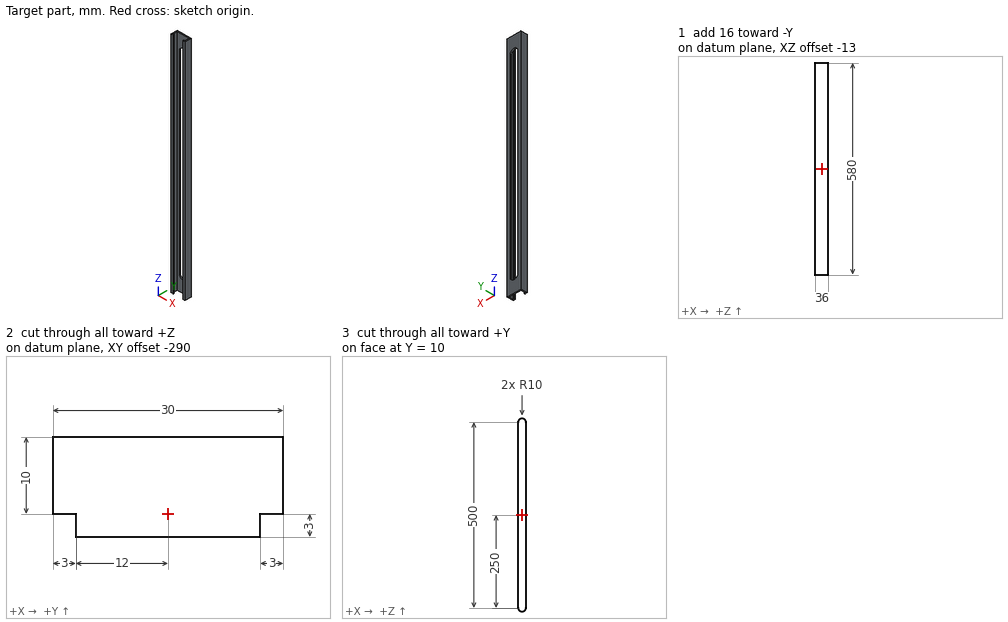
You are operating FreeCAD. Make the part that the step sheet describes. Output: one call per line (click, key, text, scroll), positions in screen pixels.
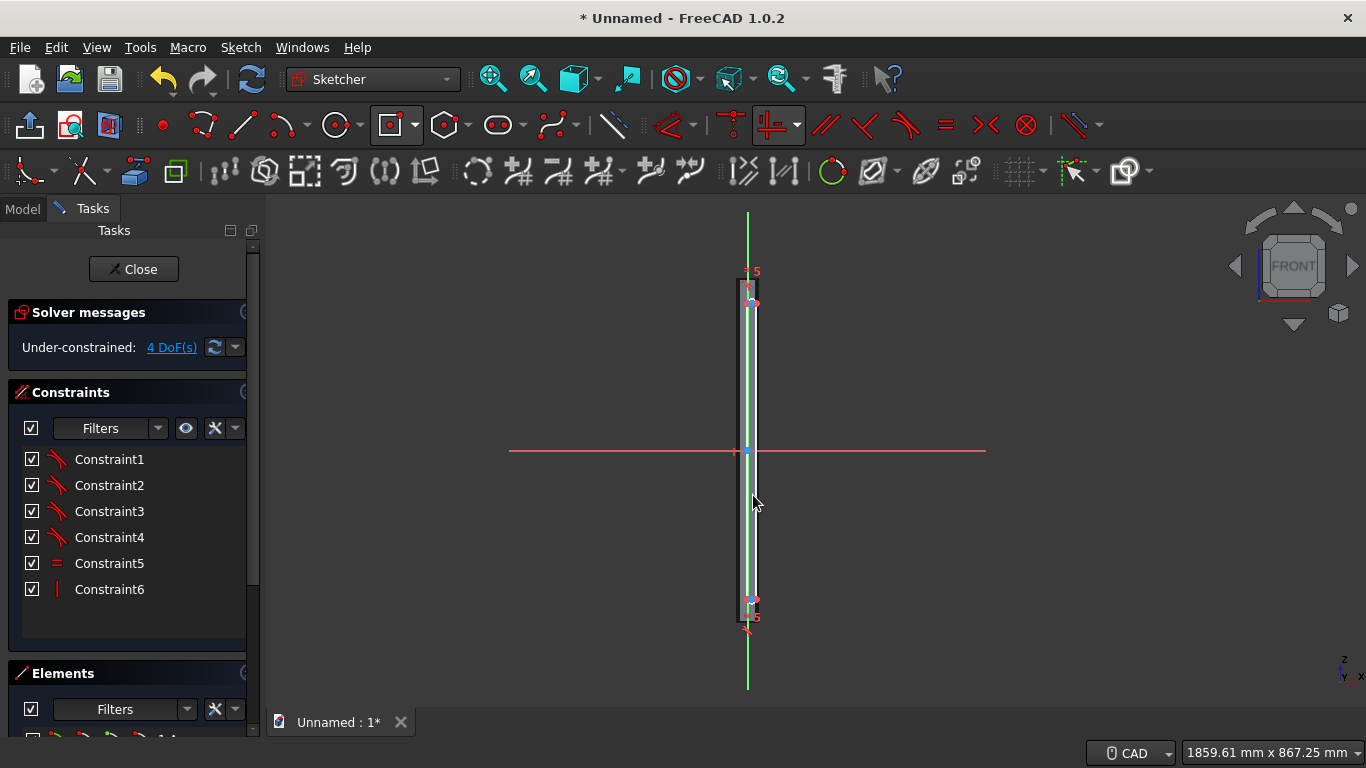
scroll(752, 599, up, 6)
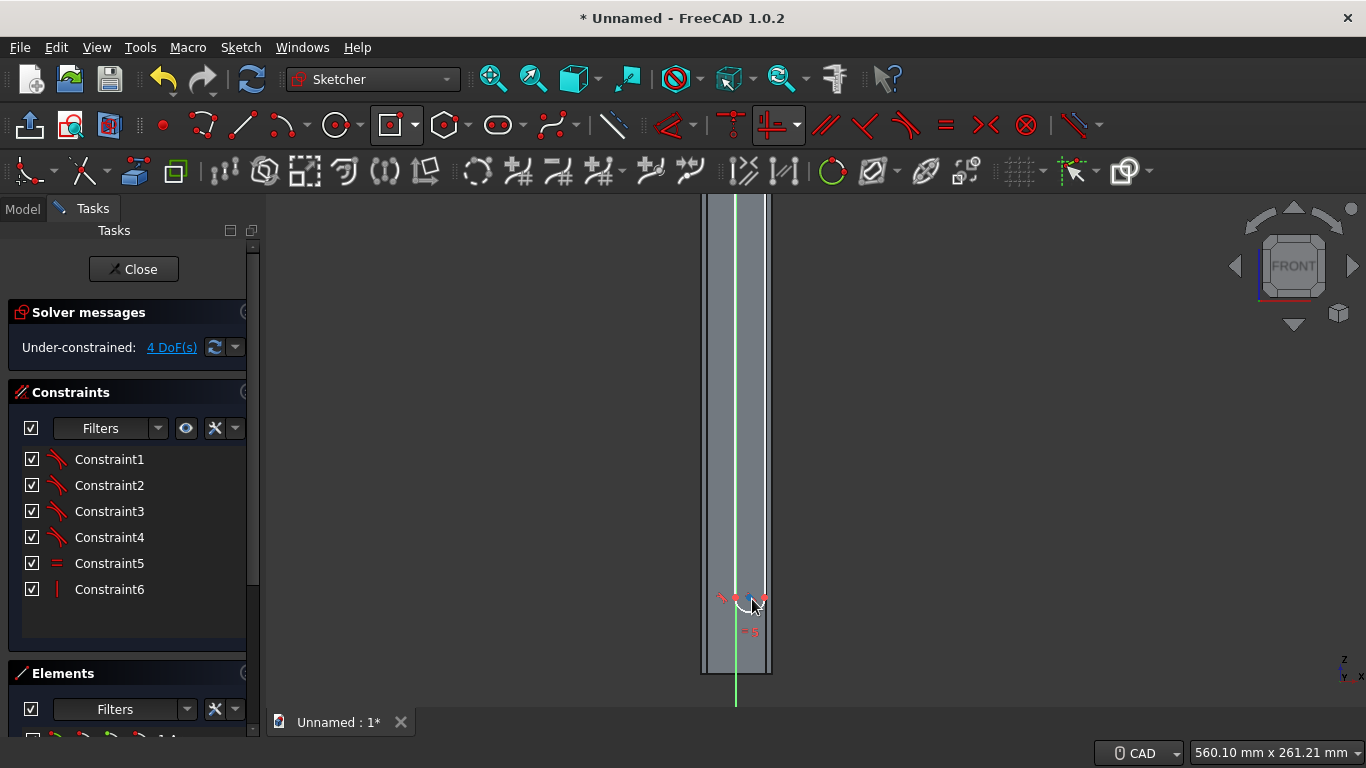
click(750, 598)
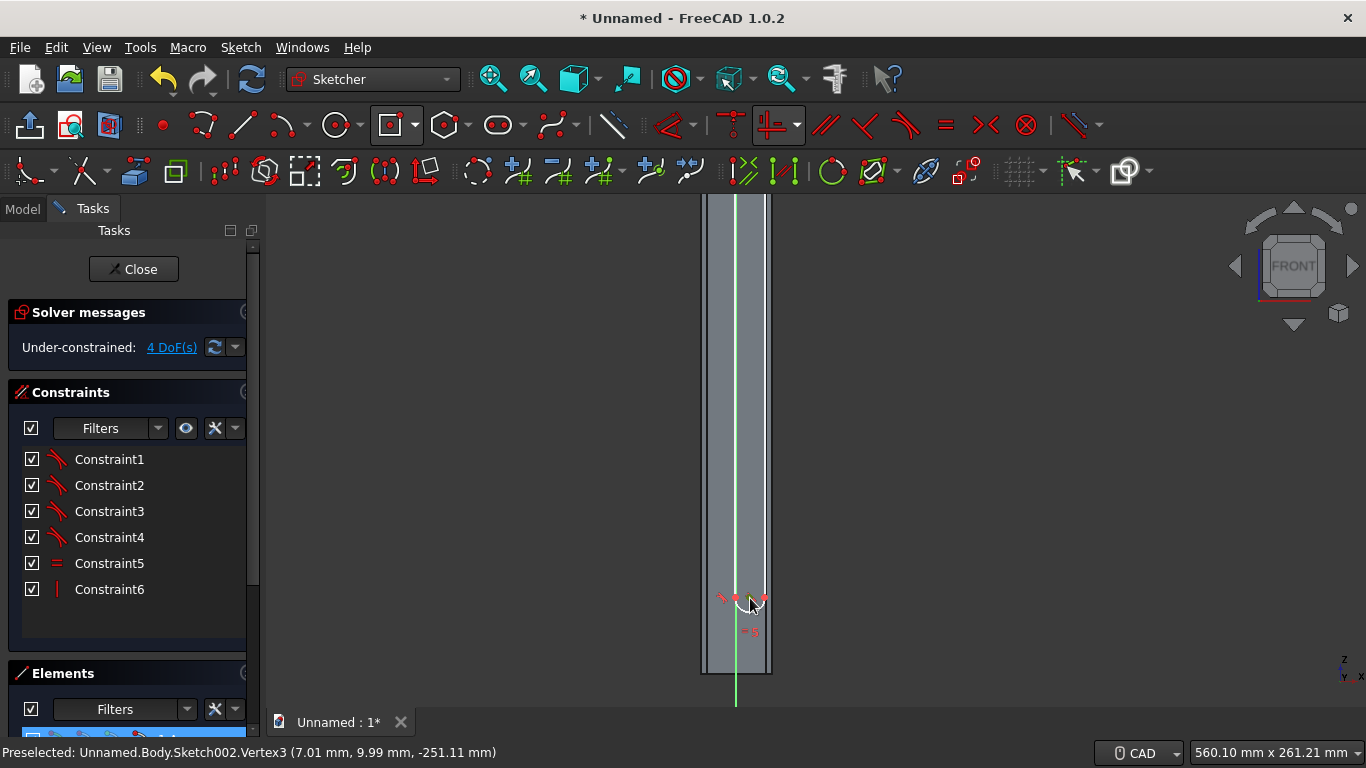
click(736, 646)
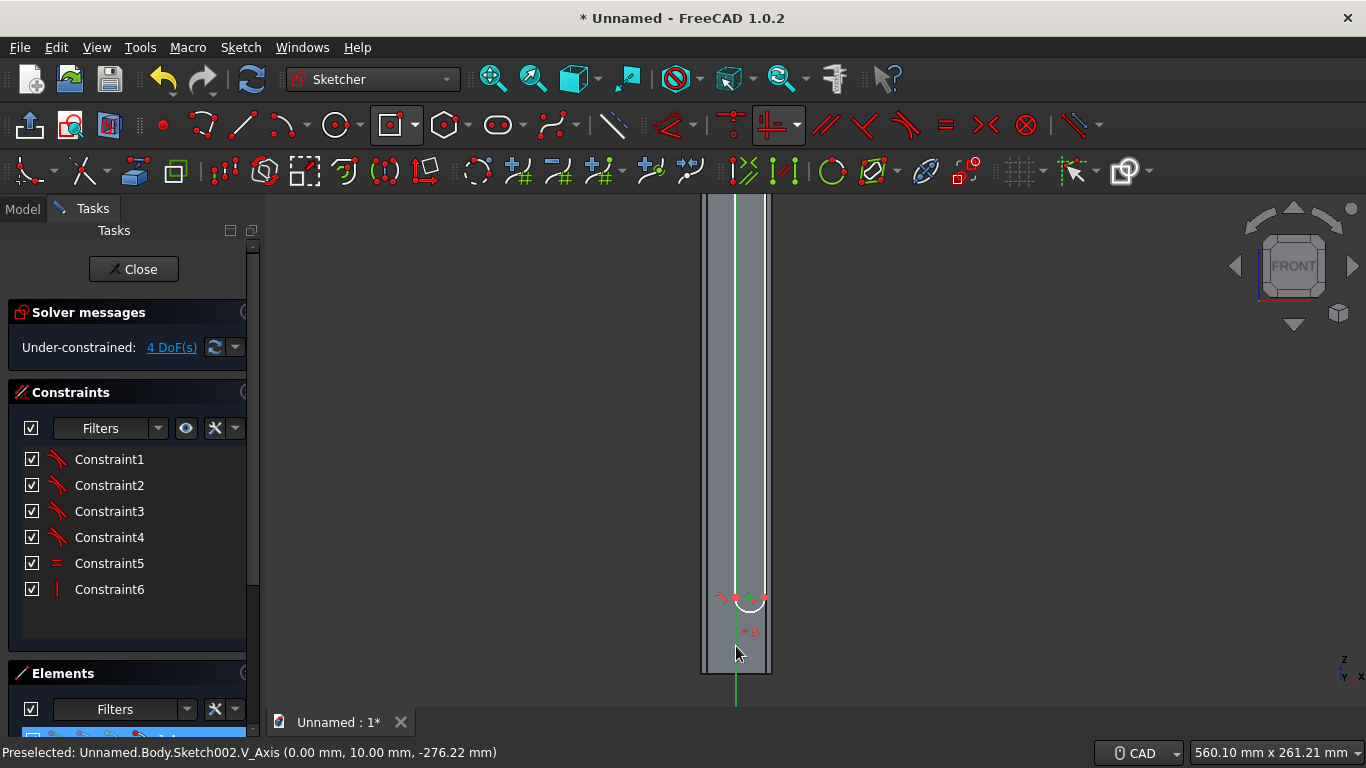
click(732, 126)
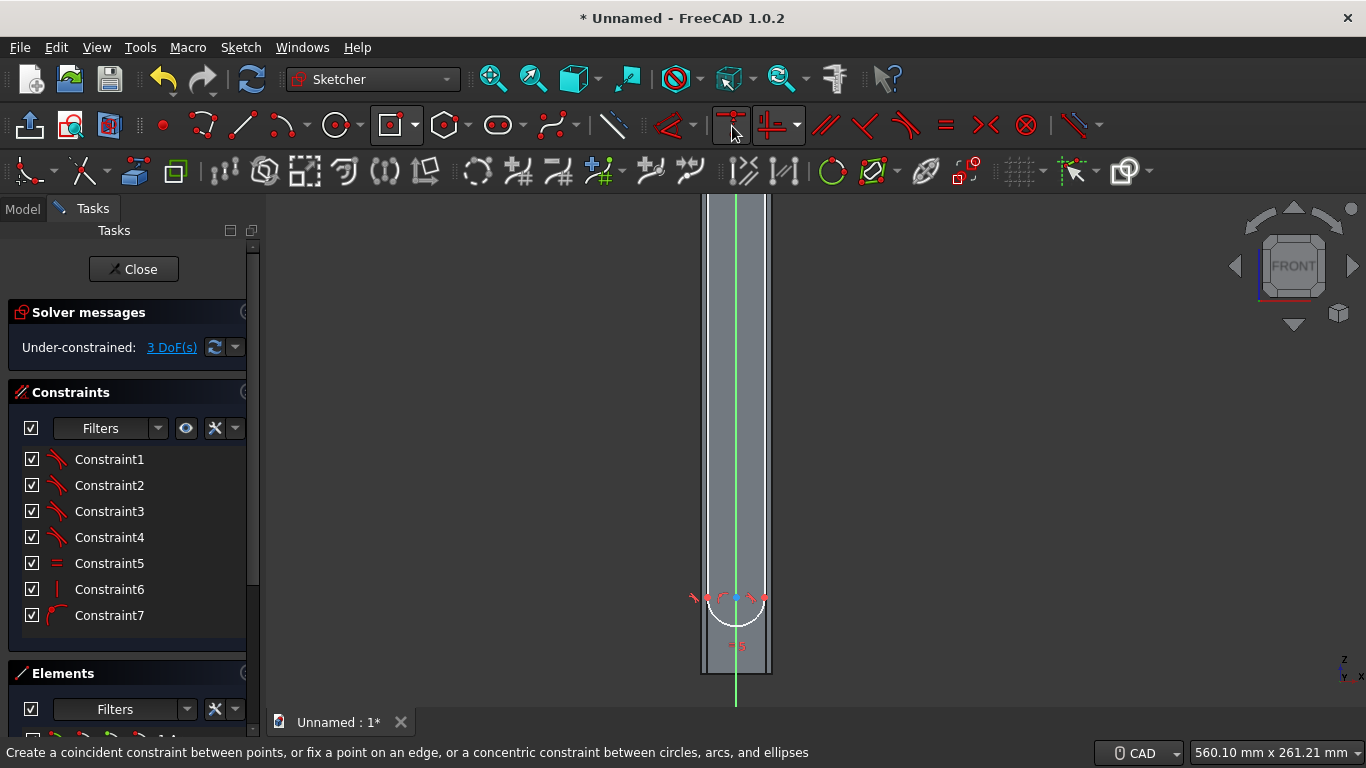
click(668, 126)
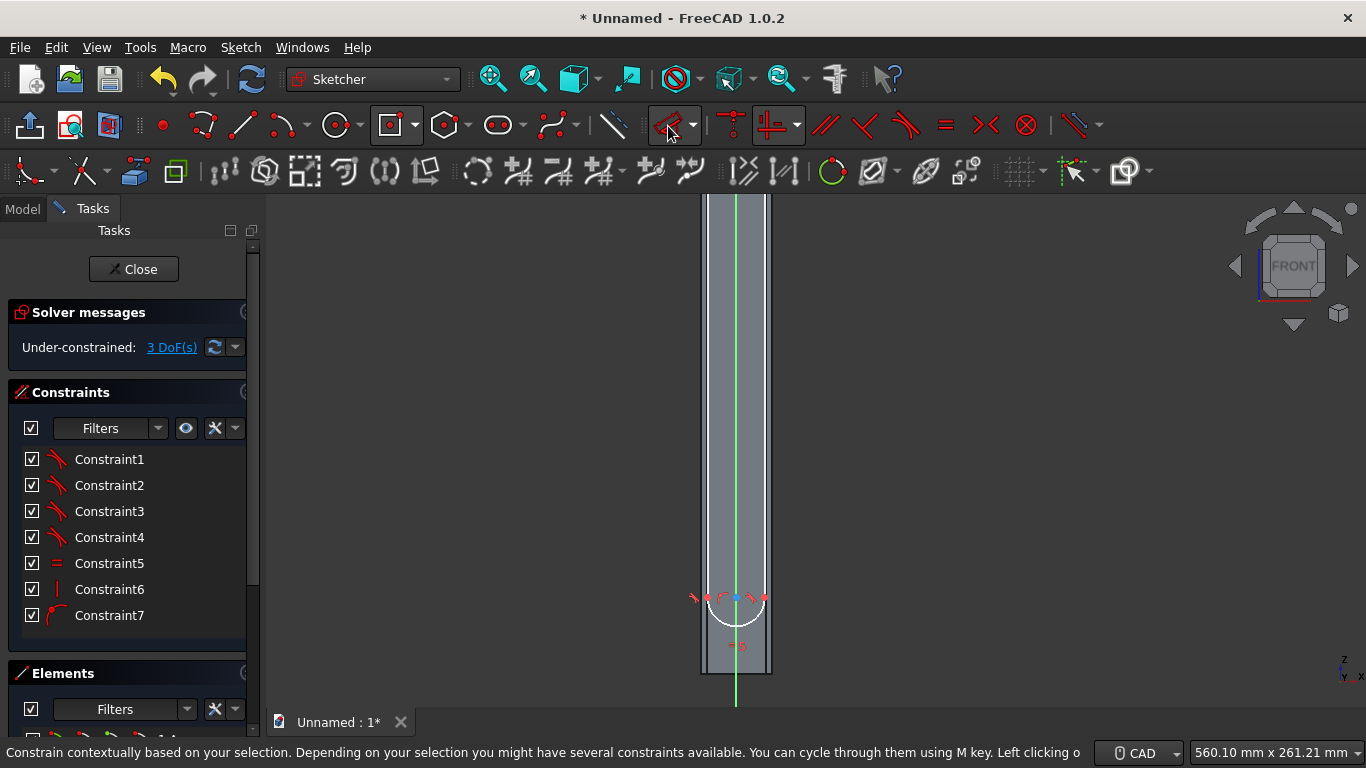
scroll(719, 621, up, 4)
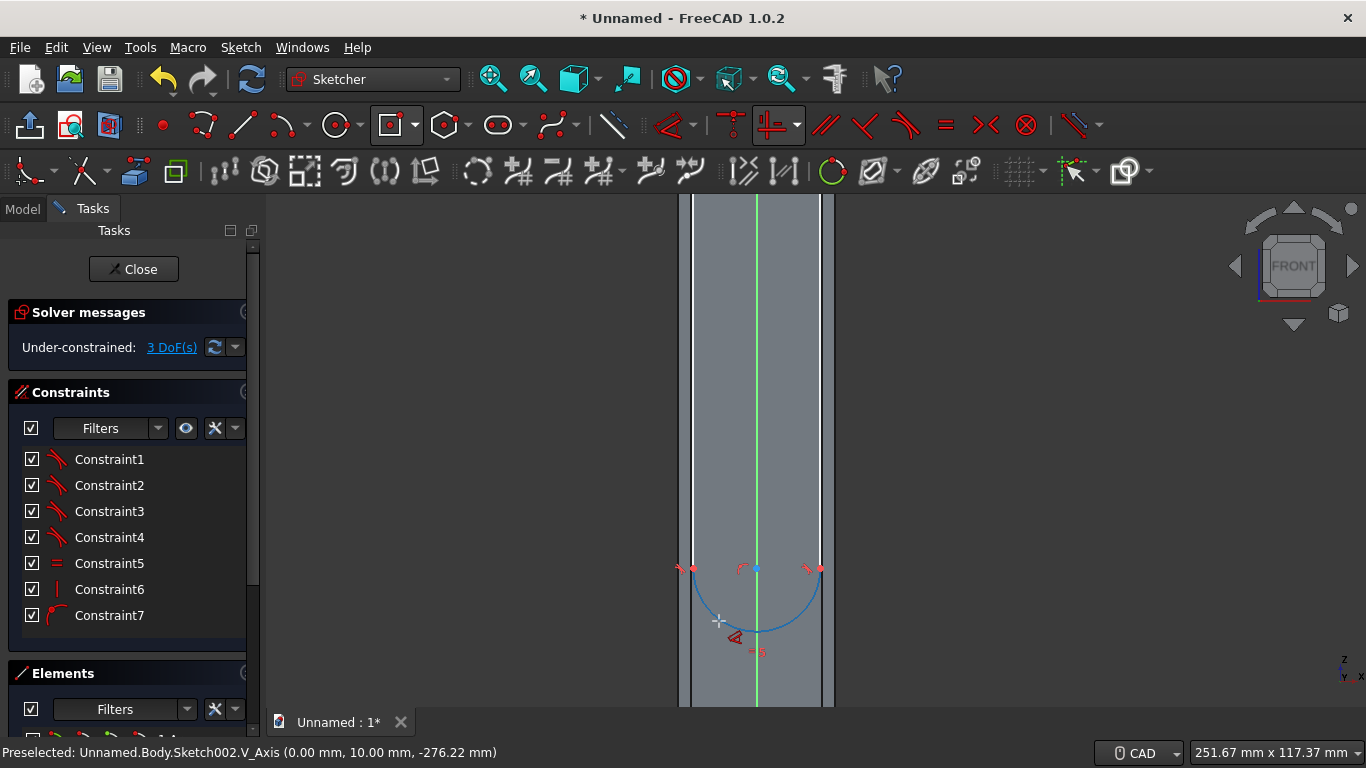
click(719, 619)
click(700, 645)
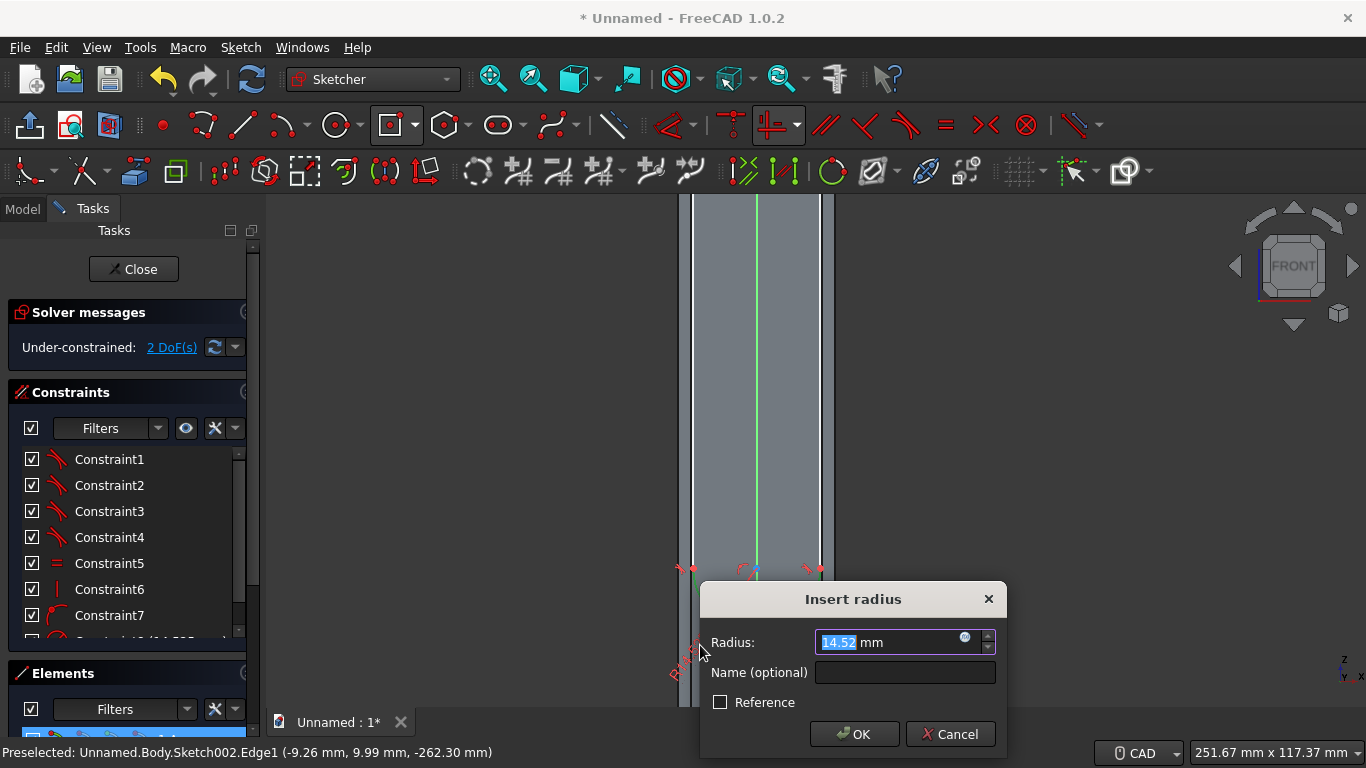
text(10)
key(Return)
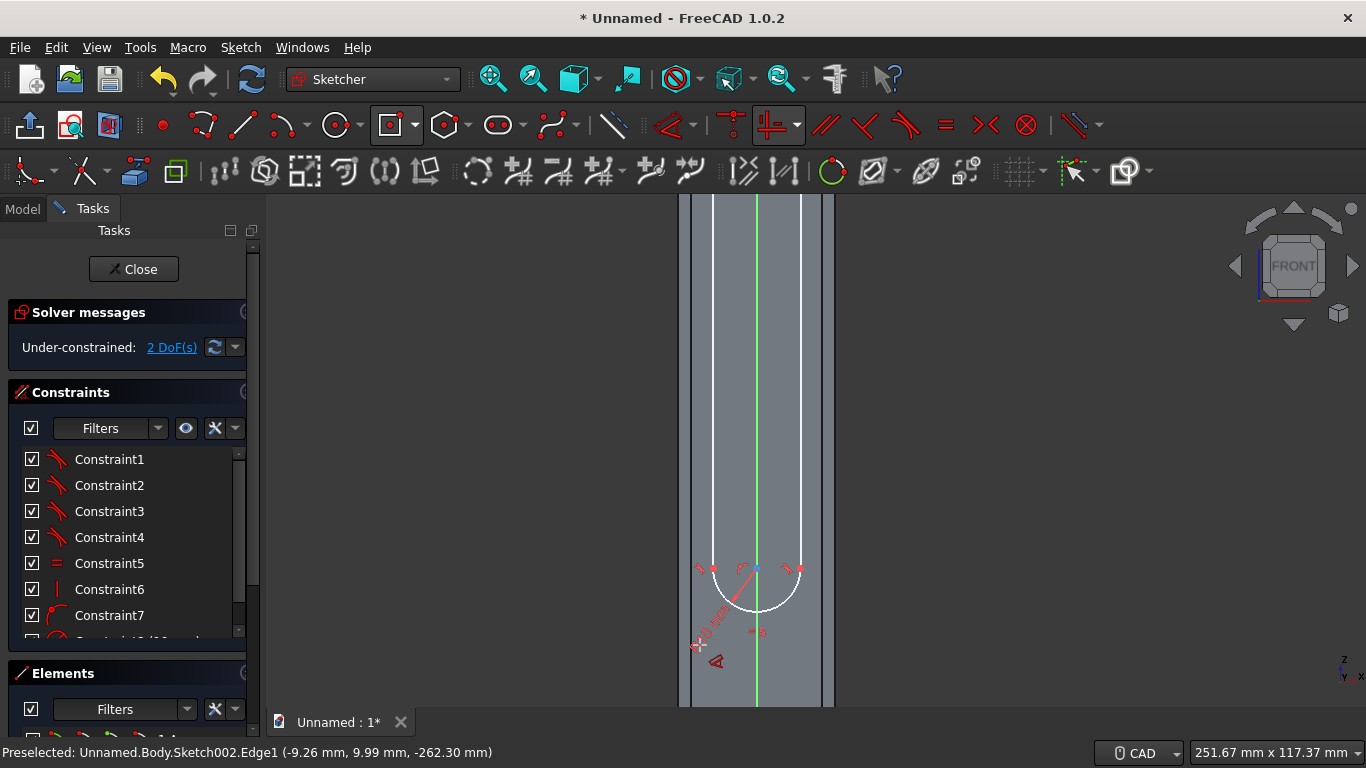
scroll(746, 604, down, 10)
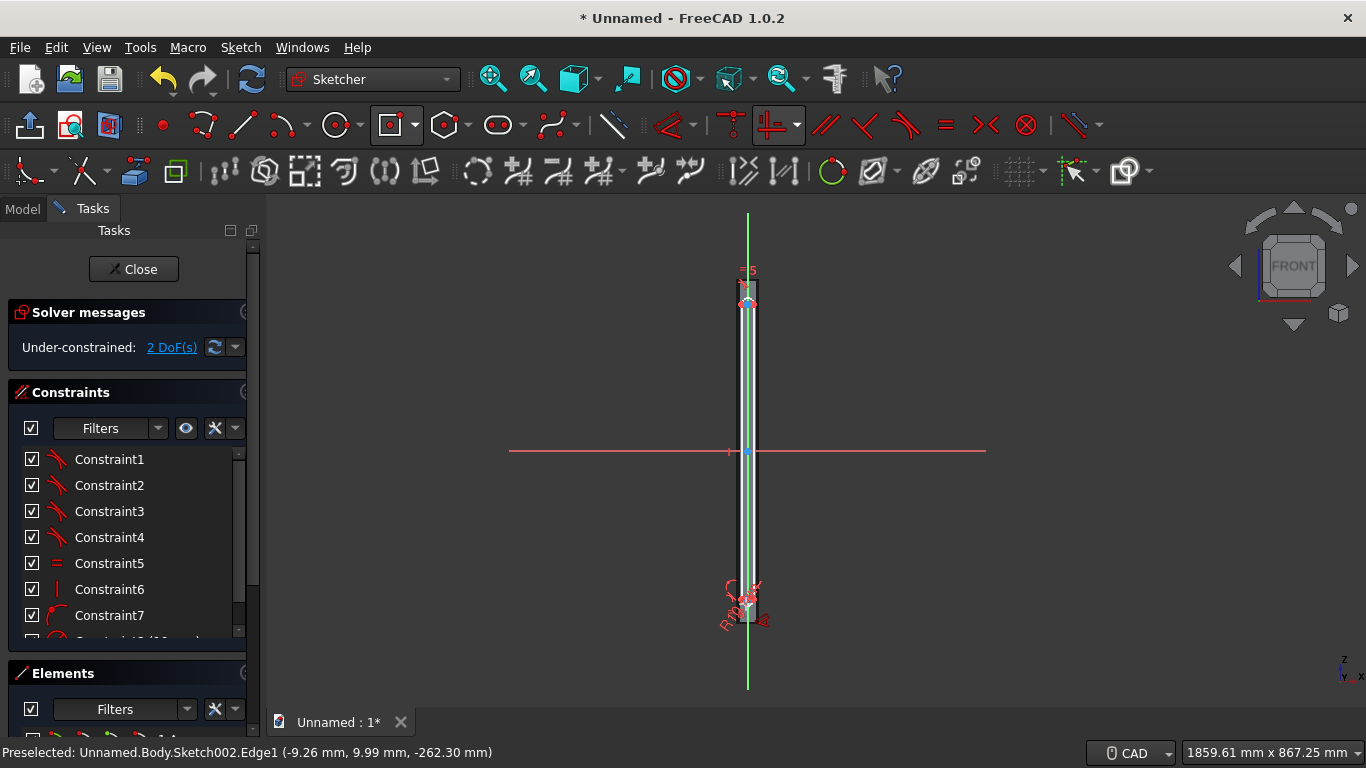
scroll(742, 511, up, 5)